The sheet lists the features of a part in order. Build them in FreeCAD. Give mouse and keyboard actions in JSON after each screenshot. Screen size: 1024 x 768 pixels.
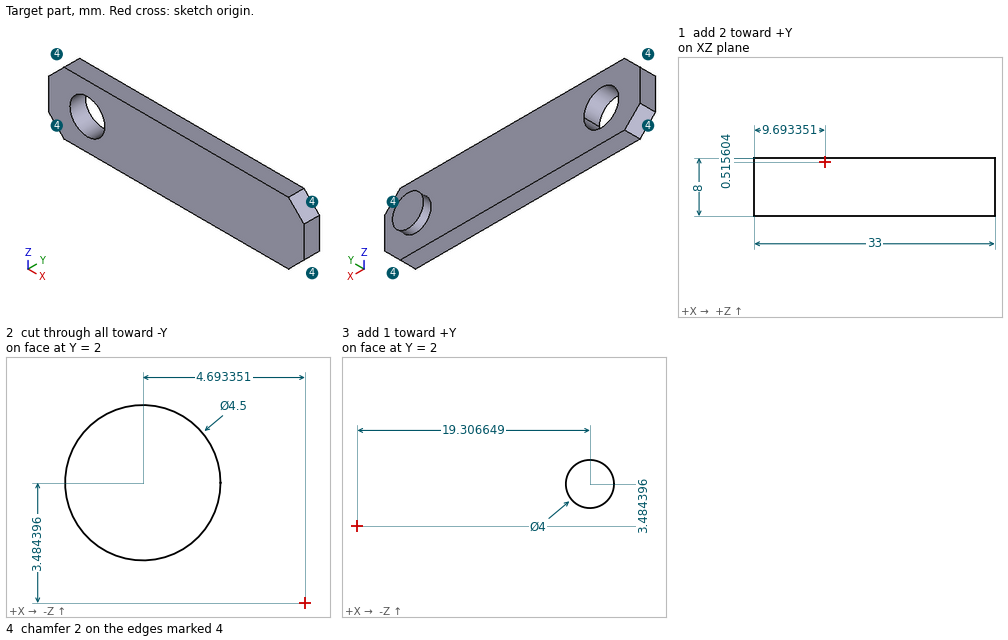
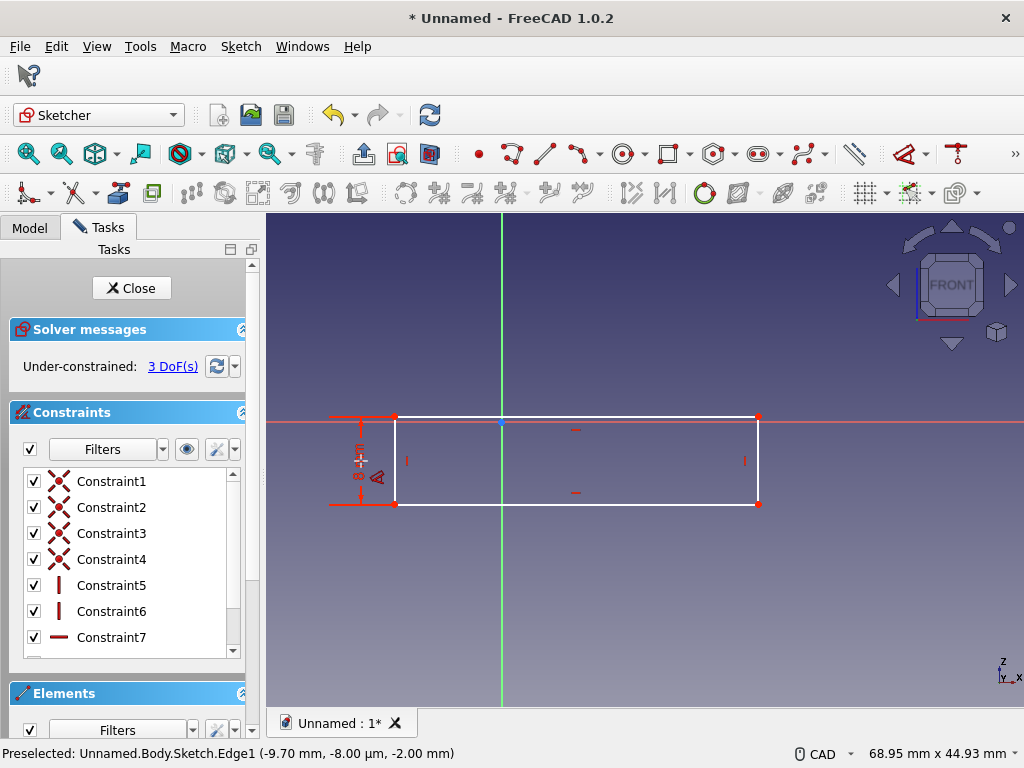
{"action": "left_click", "coordinate": [504, 505]}
{"action": "left_click", "coordinate": [576, 539]}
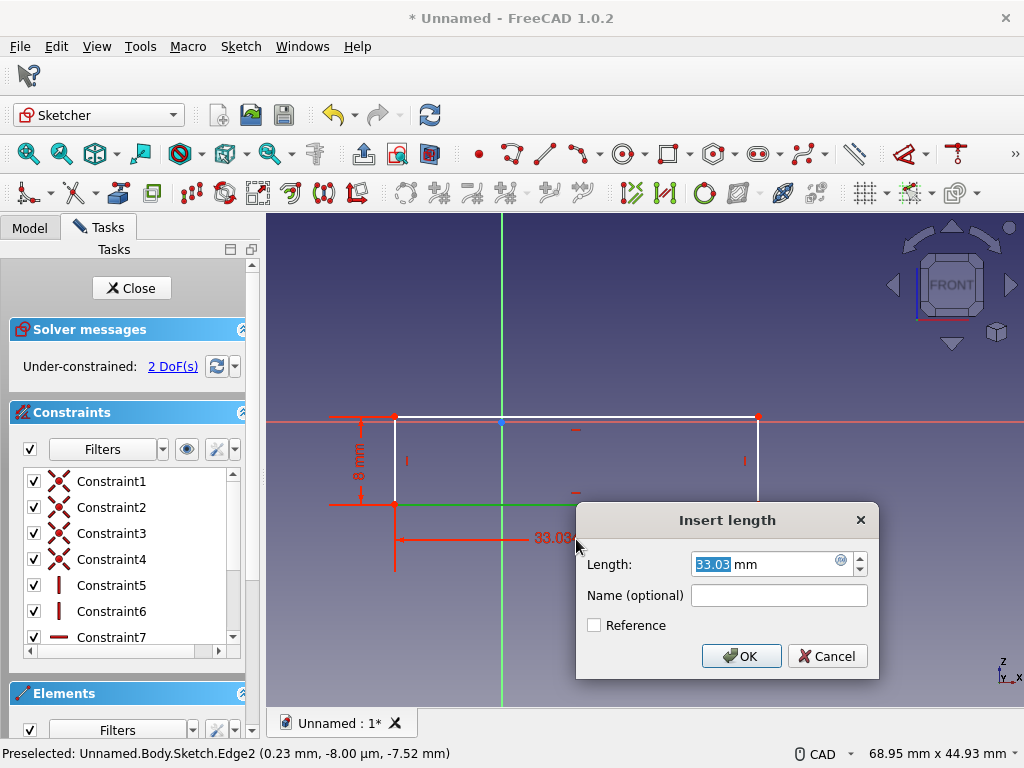
{"action": "type", "text": "33"}
{"action": "key", "text": "Return"}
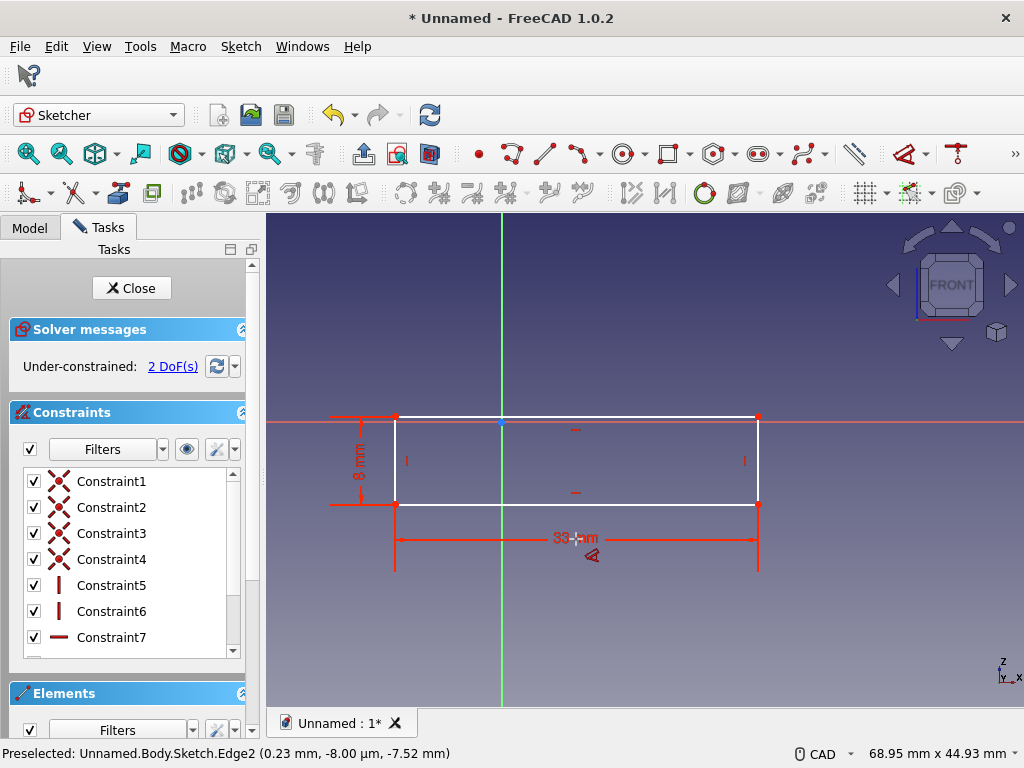
{"action": "left_click", "coordinate": [395, 417]}
{"action": "left_click", "coordinate": [448, 383]}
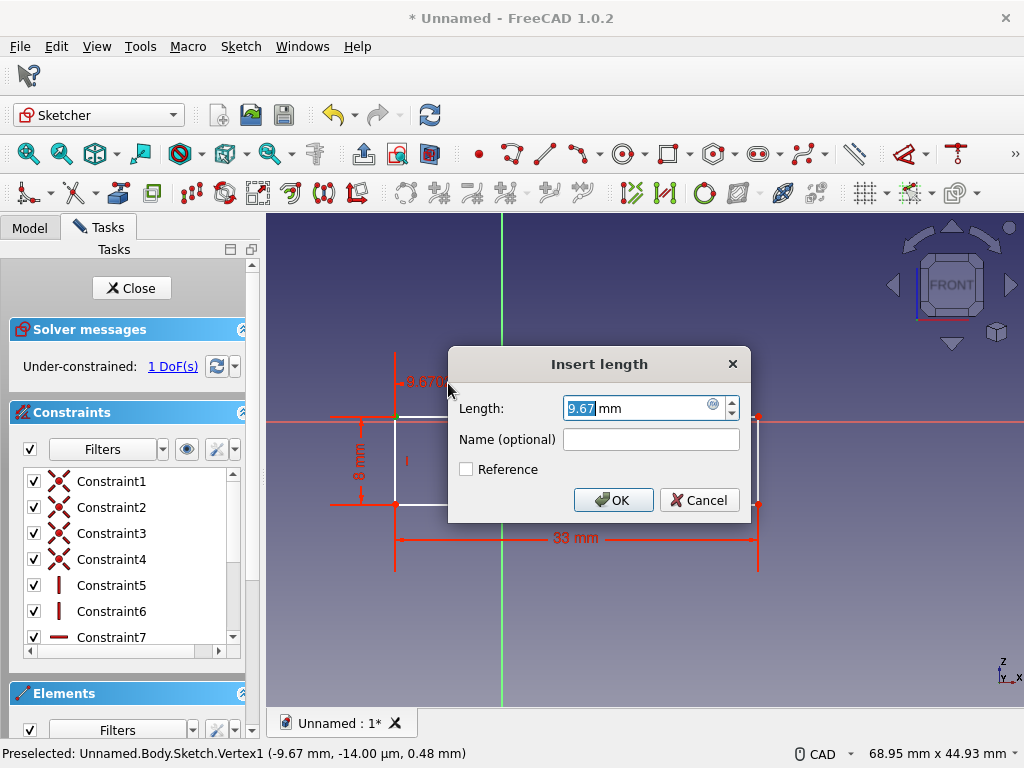
{"action": "type", "text": "9.693351"}
{"action": "key", "text": "Return"}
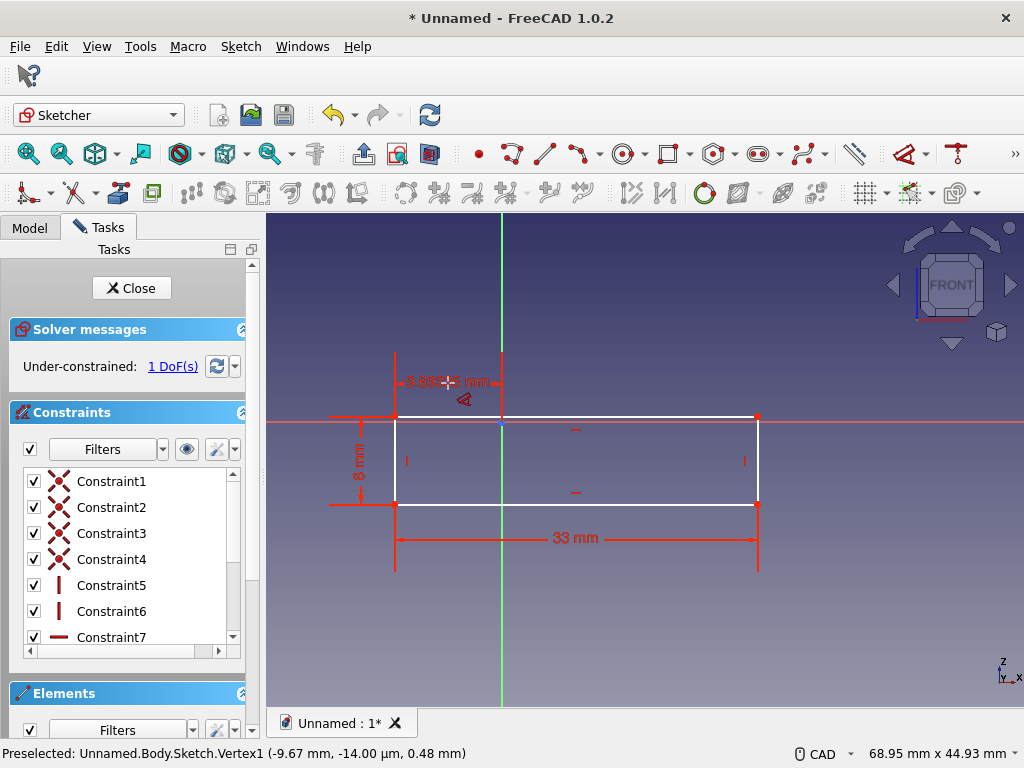
{"action": "scroll", "coordinate": [395, 417], "scroll_direction": "up", "scroll_amount": 10}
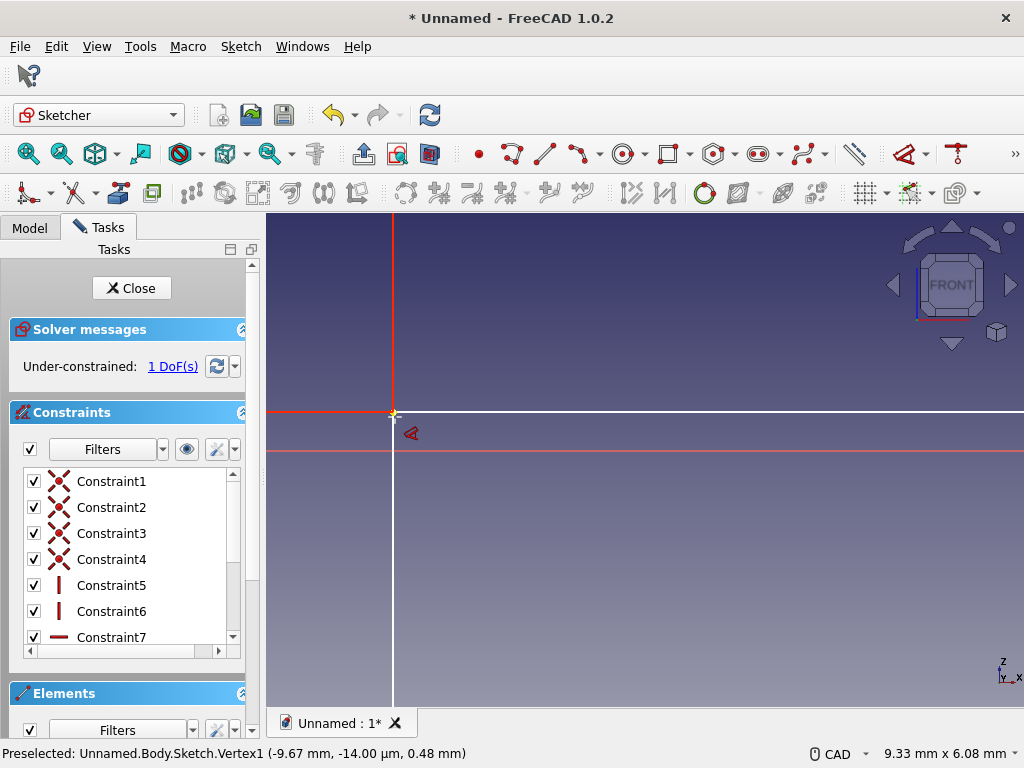
{"action": "left_click", "coordinate": [393, 412]}
{"action": "left_click", "coordinate": [359, 432]}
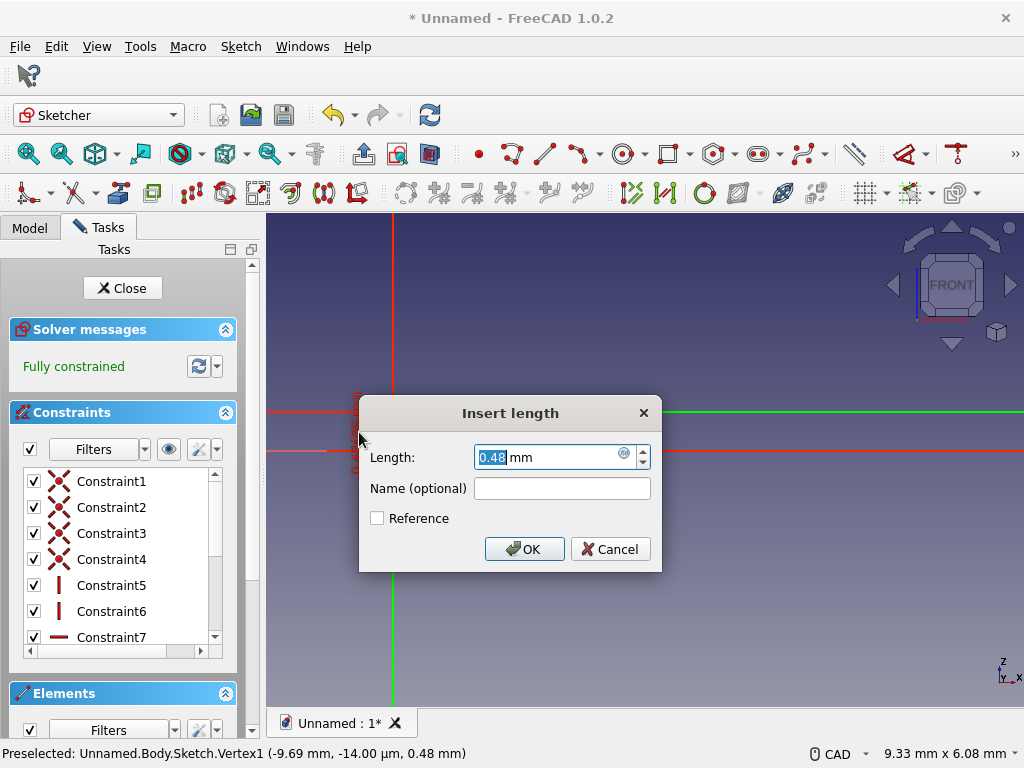
{"action": "type", "text": "0.515604"}
{"action": "key", "text": "Return"}
{"action": "key", "text": "Escape"}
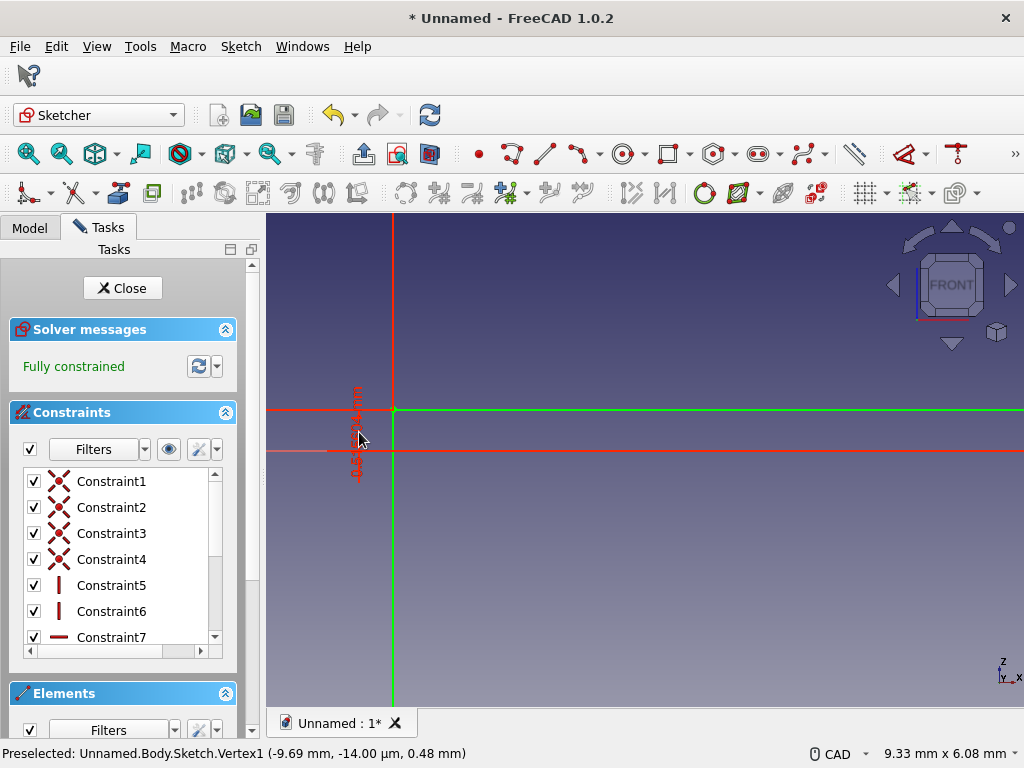
{"action": "left_click", "coordinate": [123, 288]}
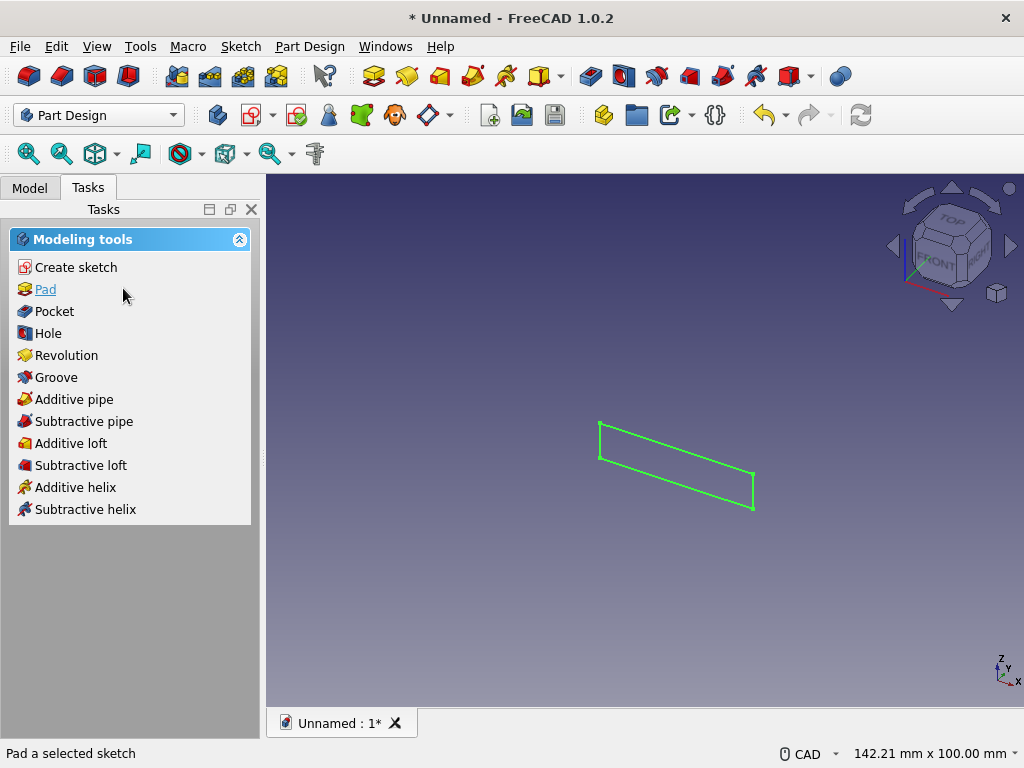
{"action": "left_click", "coordinate": [374, 76]}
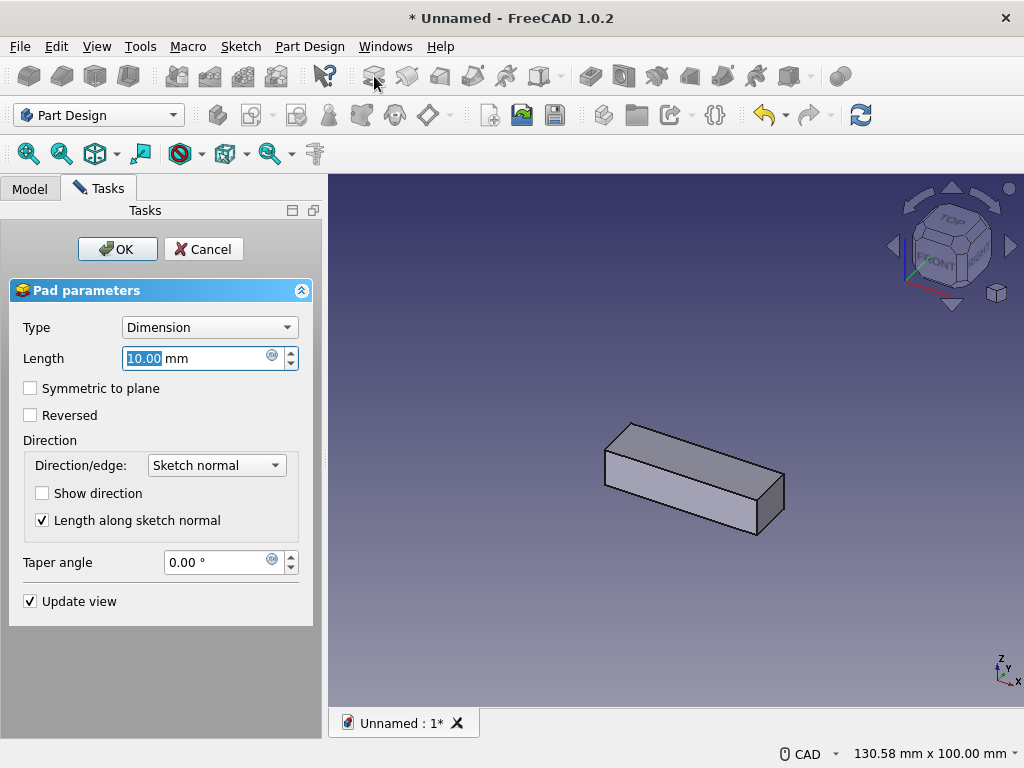
{"action": "type", "text": "2"}
{"action": "key", "text": "Tab"}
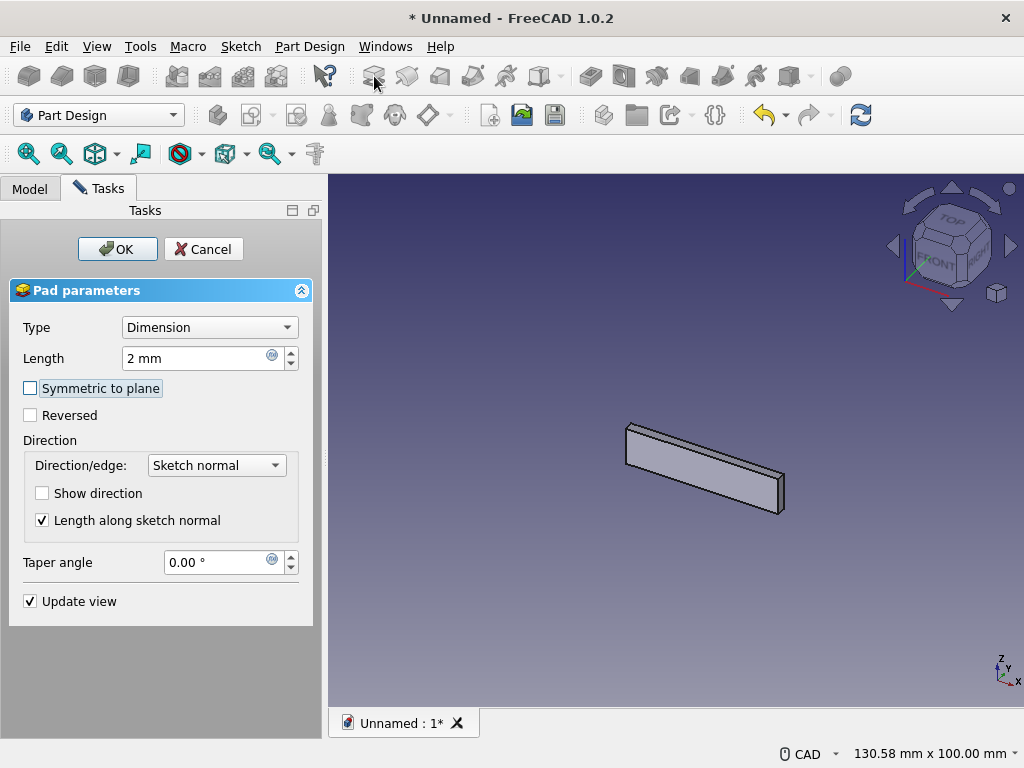
{"action": "left_click", "coordinate": [31, 415]}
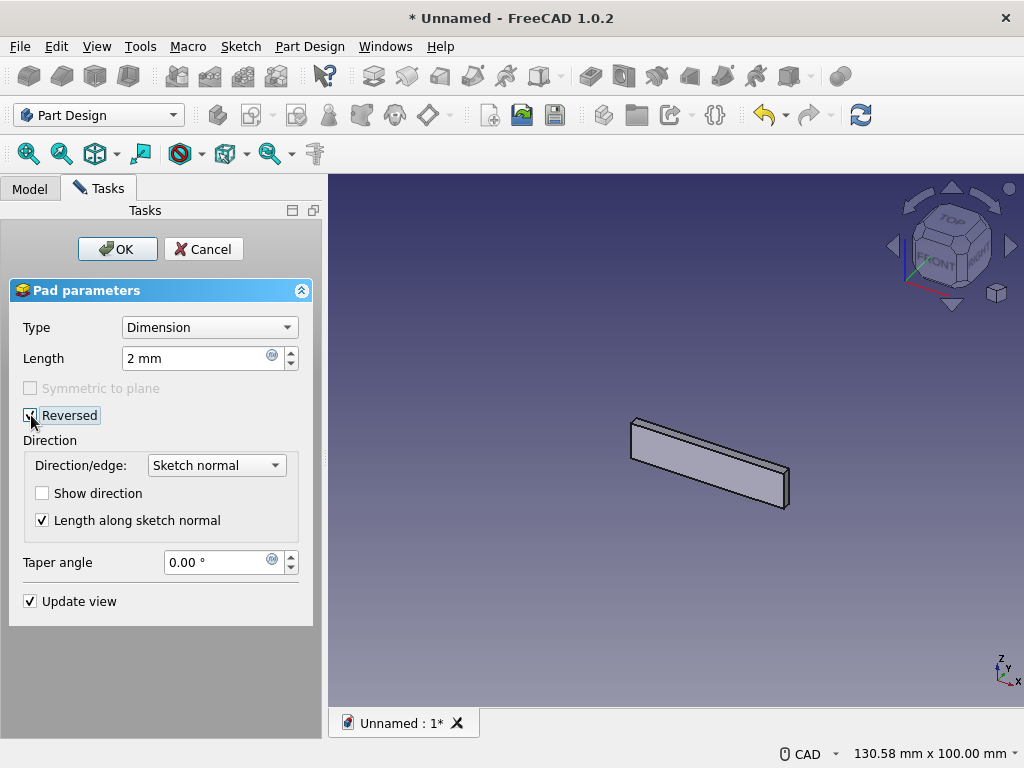
{"action": "left_click", "coordinate": [118, 249]}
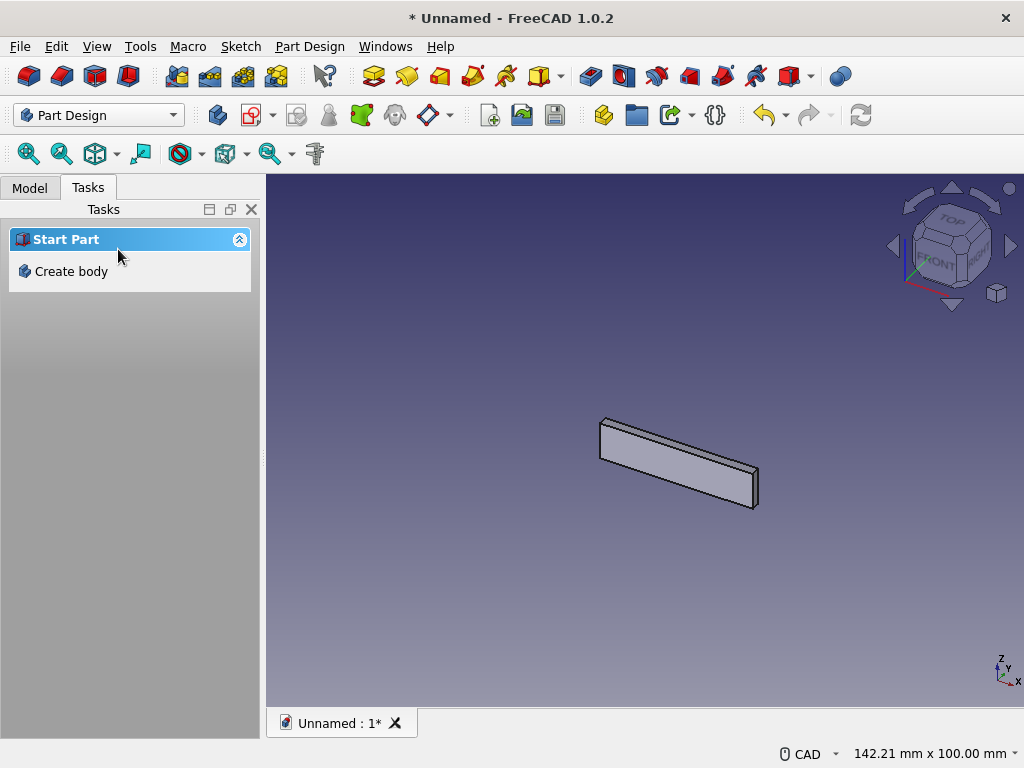
{"action": "left_click", "coordinate": [29, 154]}